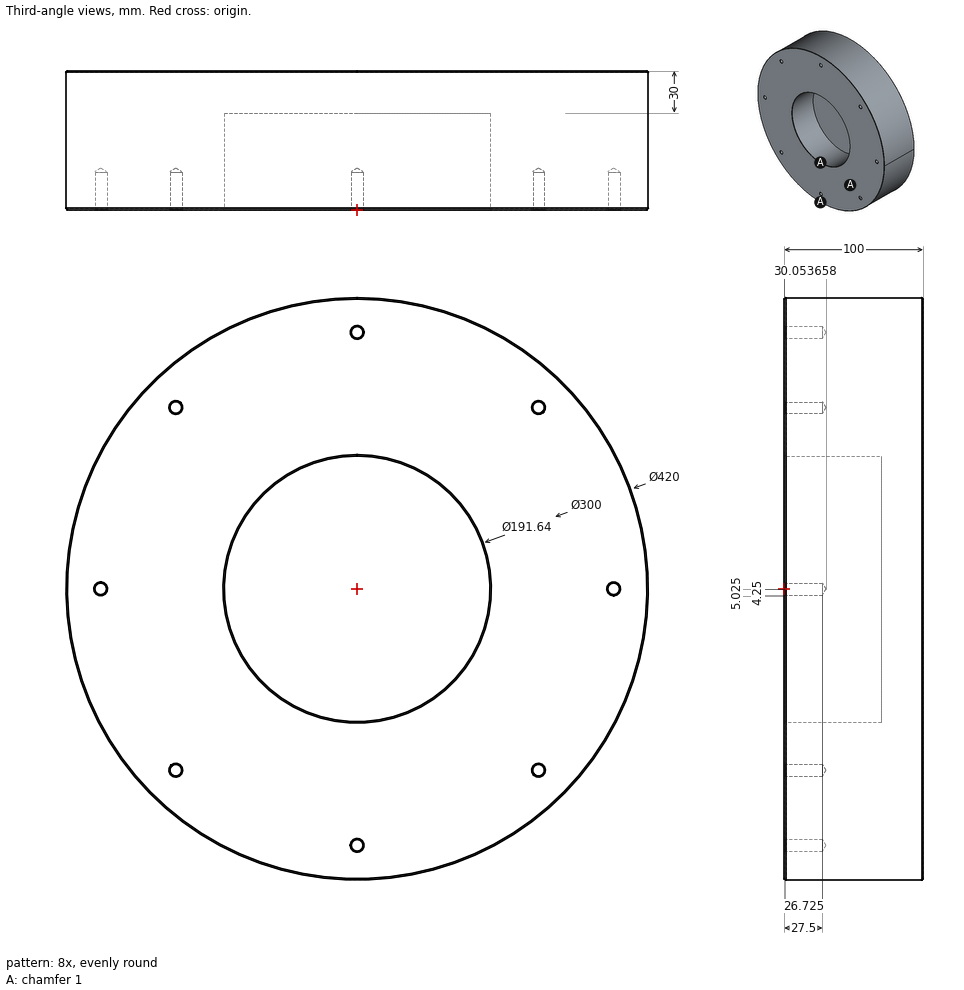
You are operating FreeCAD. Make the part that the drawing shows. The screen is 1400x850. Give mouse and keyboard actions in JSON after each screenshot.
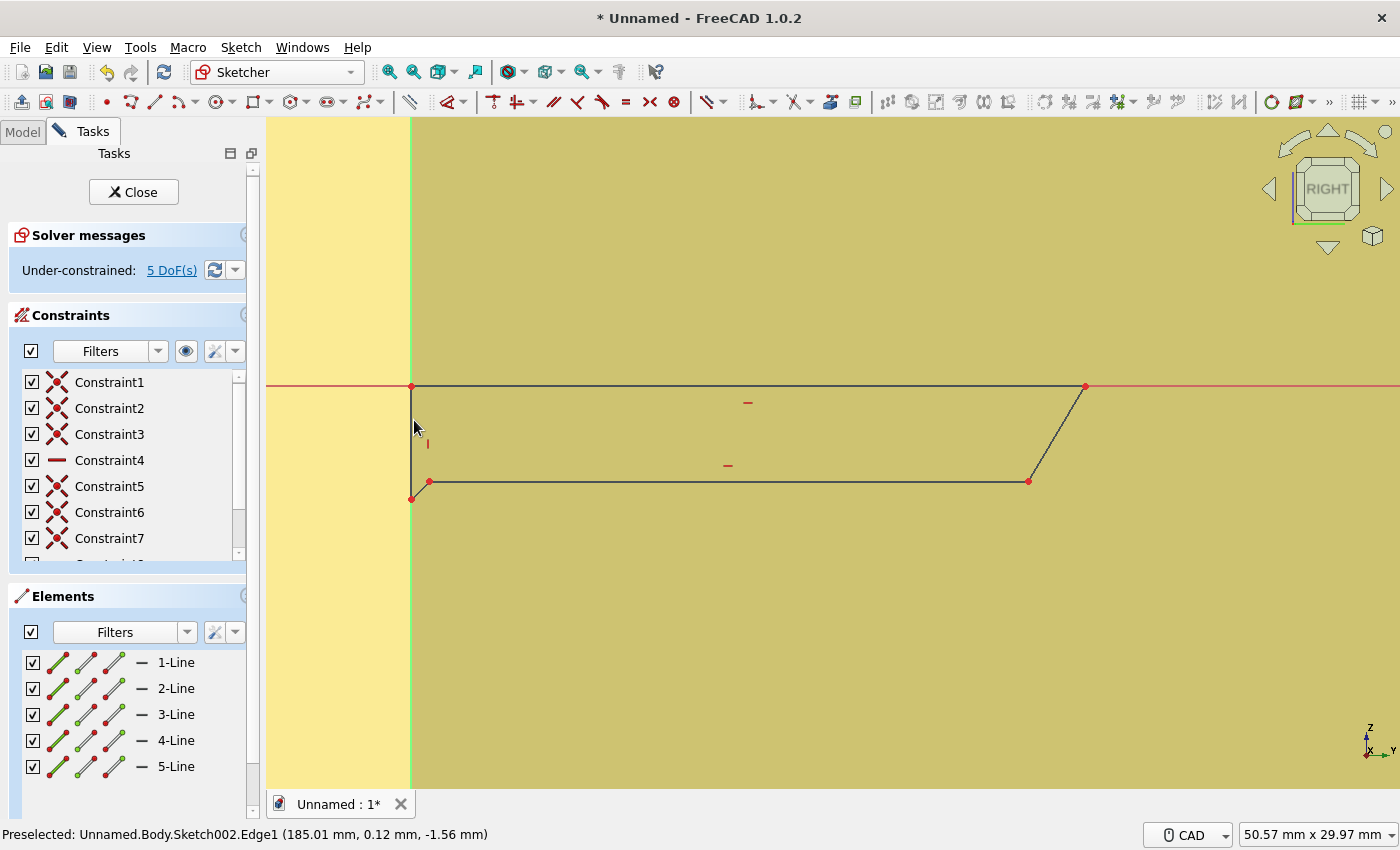
{"action": "left_click", "coordinate": [411, 420]}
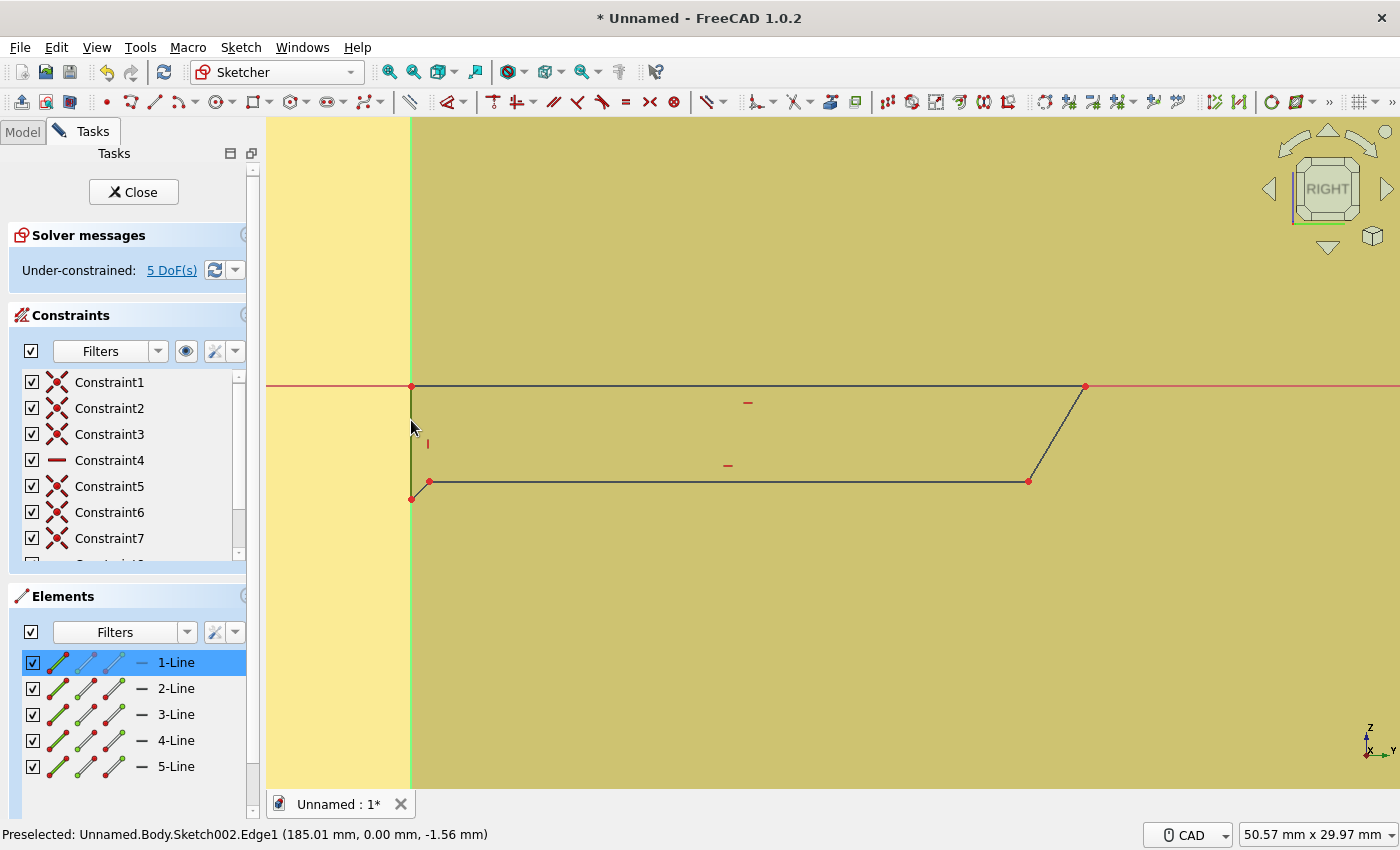
{"action": "left_click", "coordinate": [466, 102]}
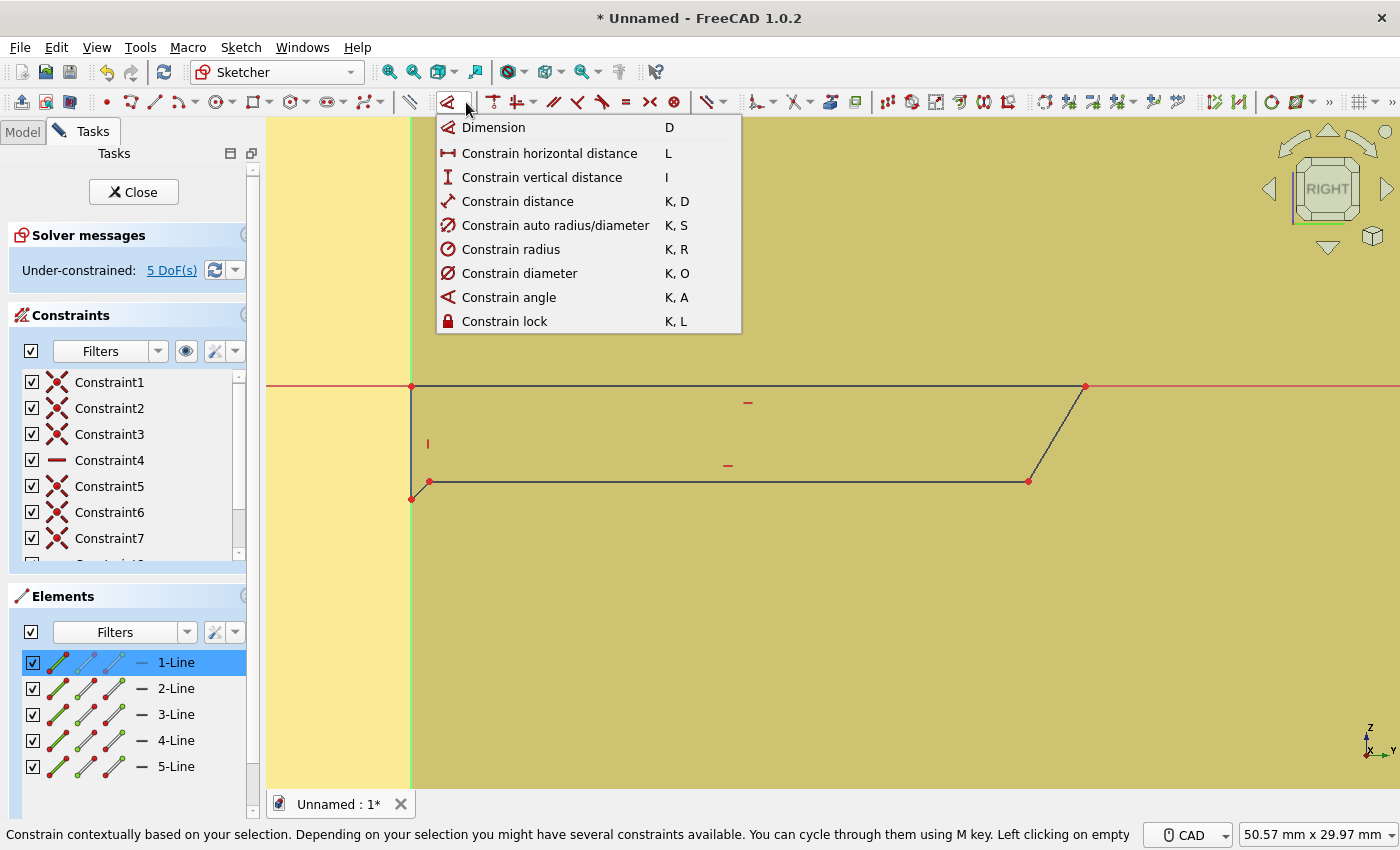
{"action": "left_click", "coordinate": [589, 177]}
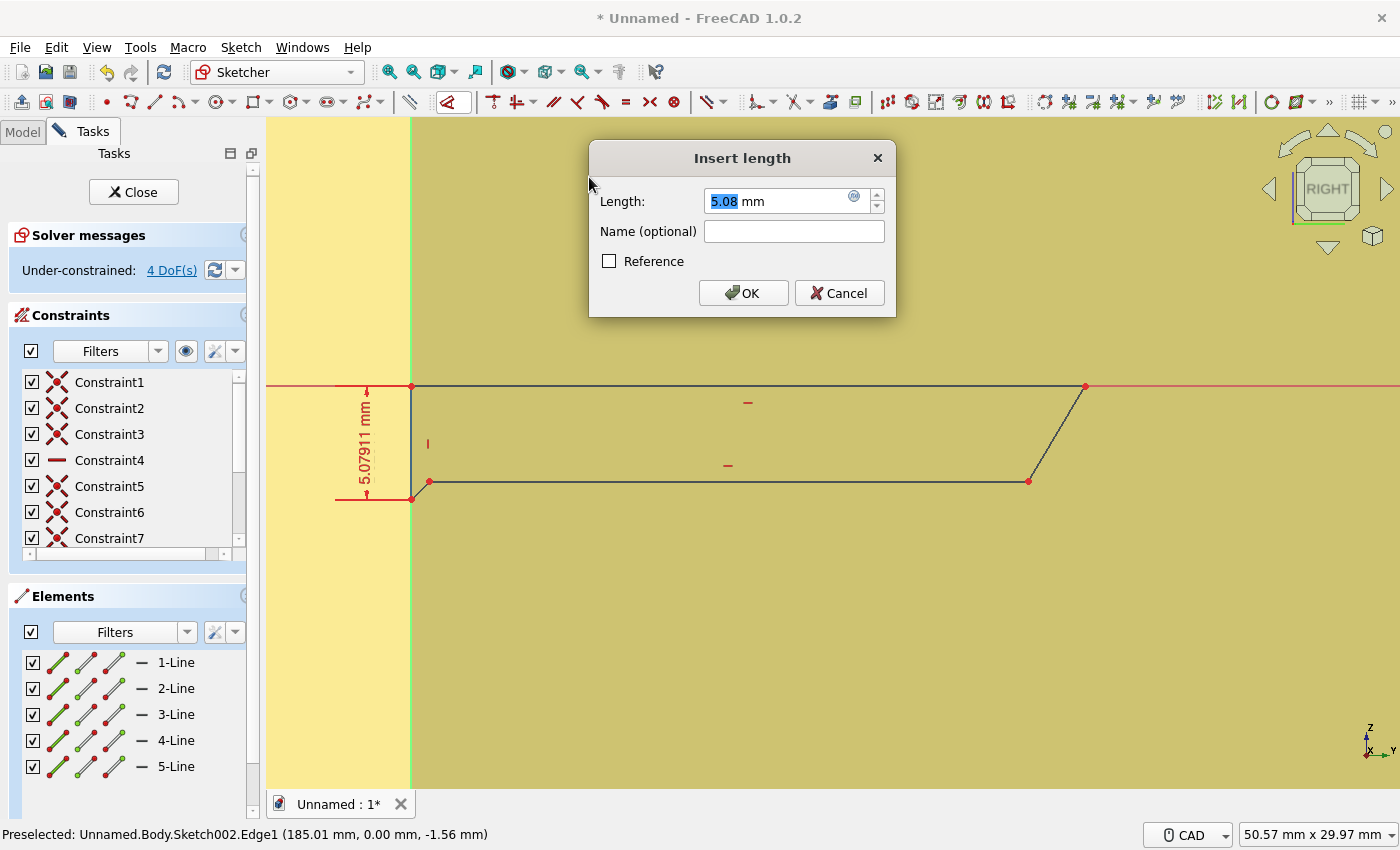
{"action": "type", "text": "5.025"}
{"action": "key", "text": "Return"}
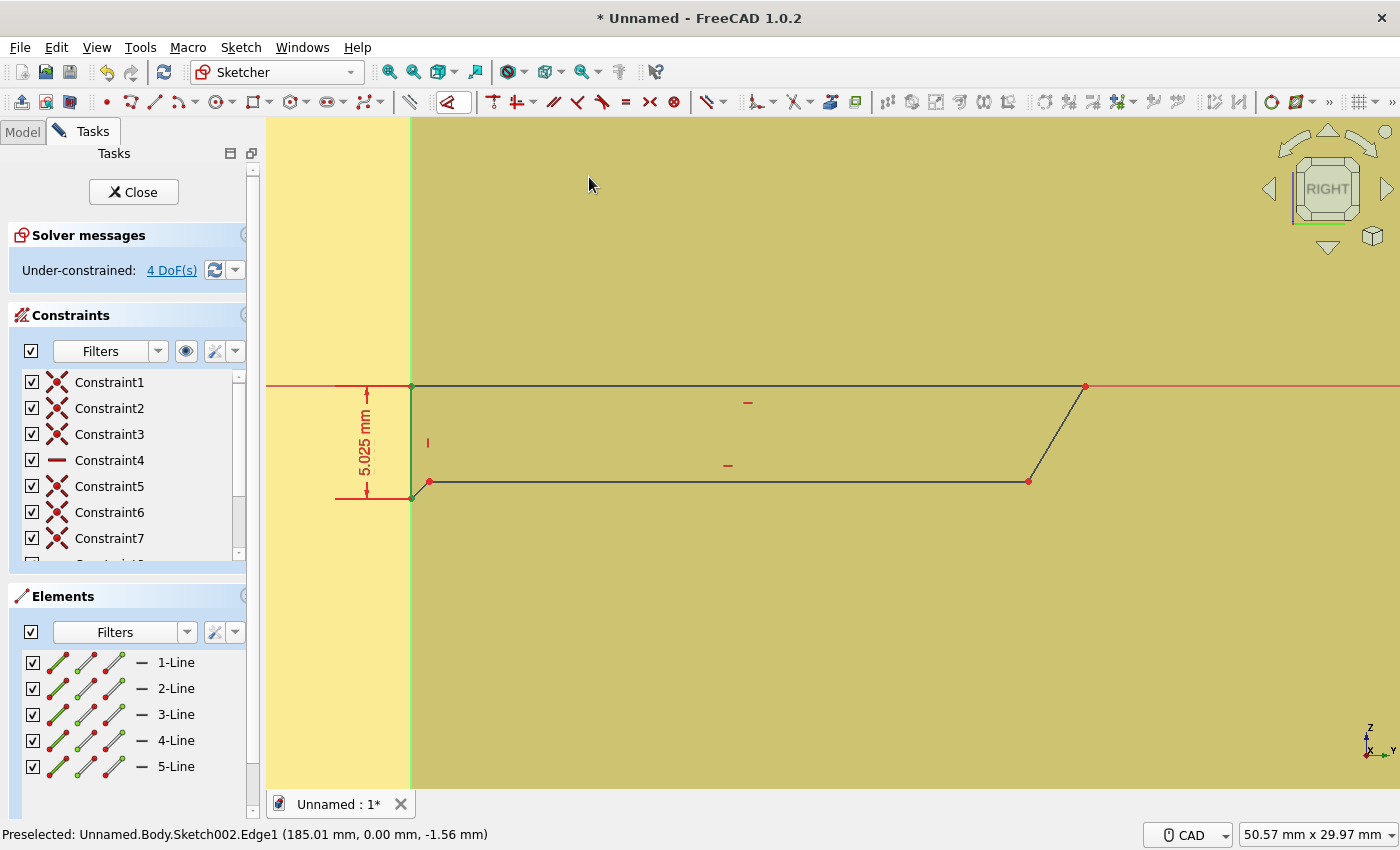
{"action": "left_click", "coordinate": [429, 482]}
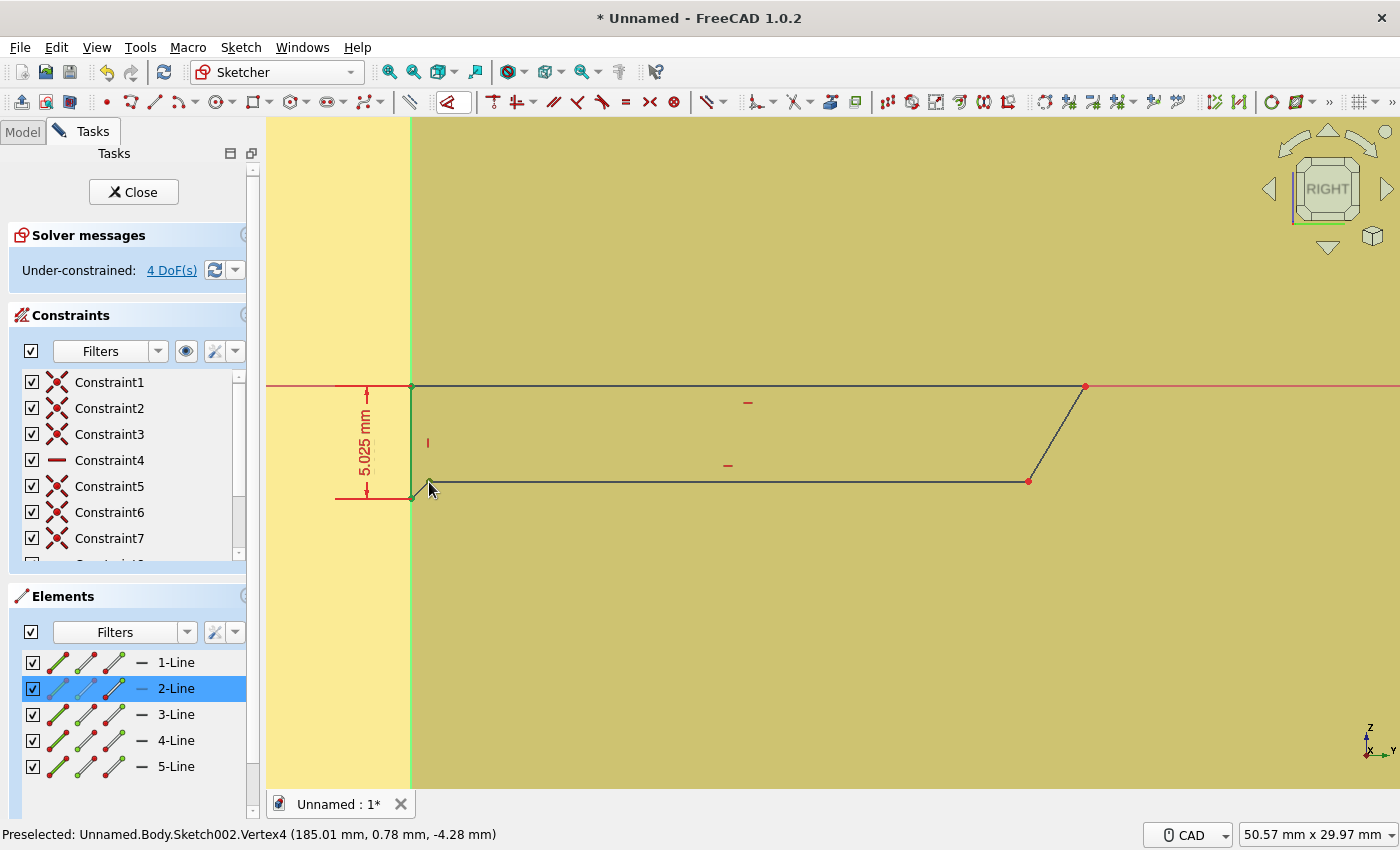
{"action": "key", "text": "i"}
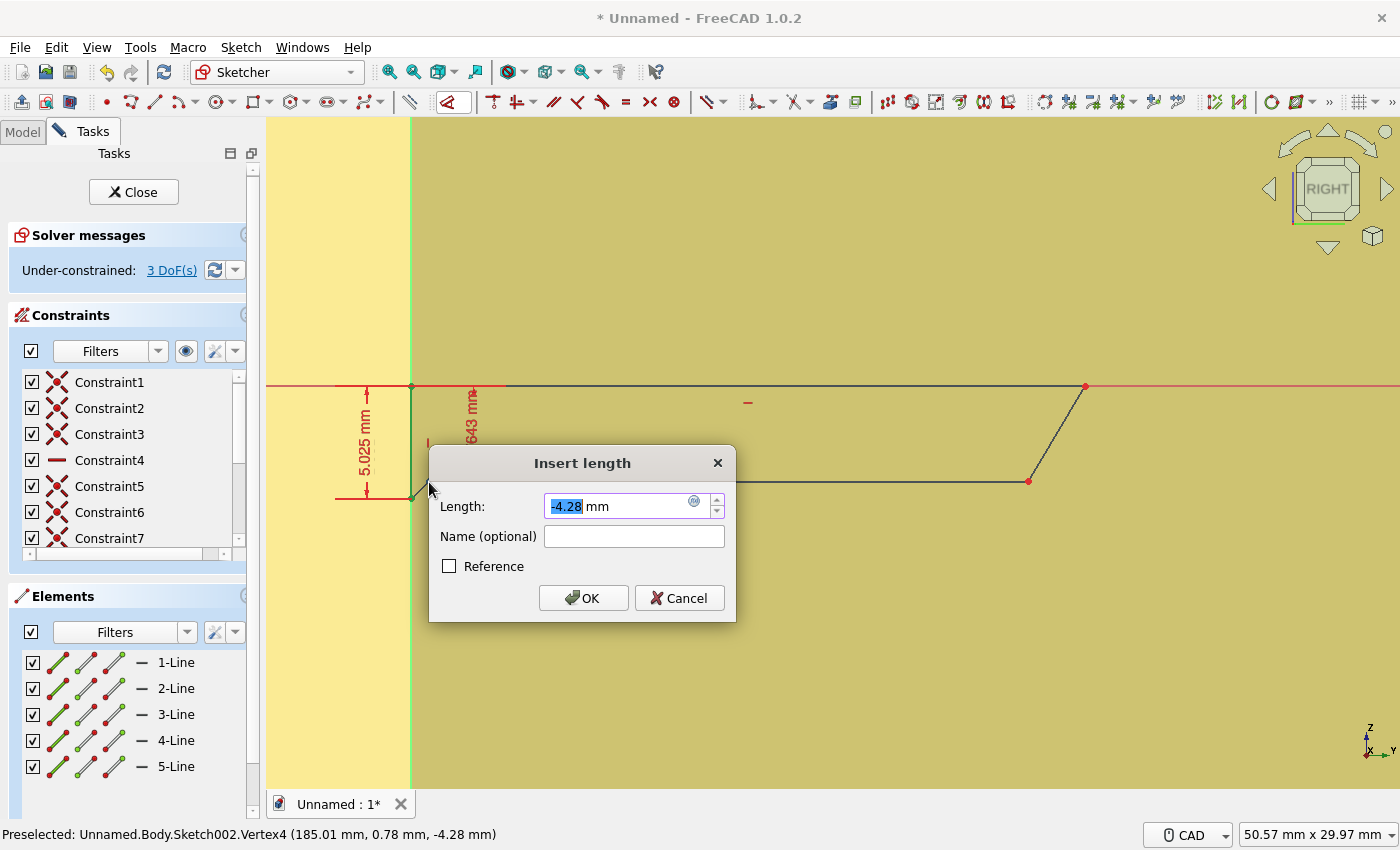
{"action": "type", "text": "-4.25"}
{"action": "key", "text": "Return"}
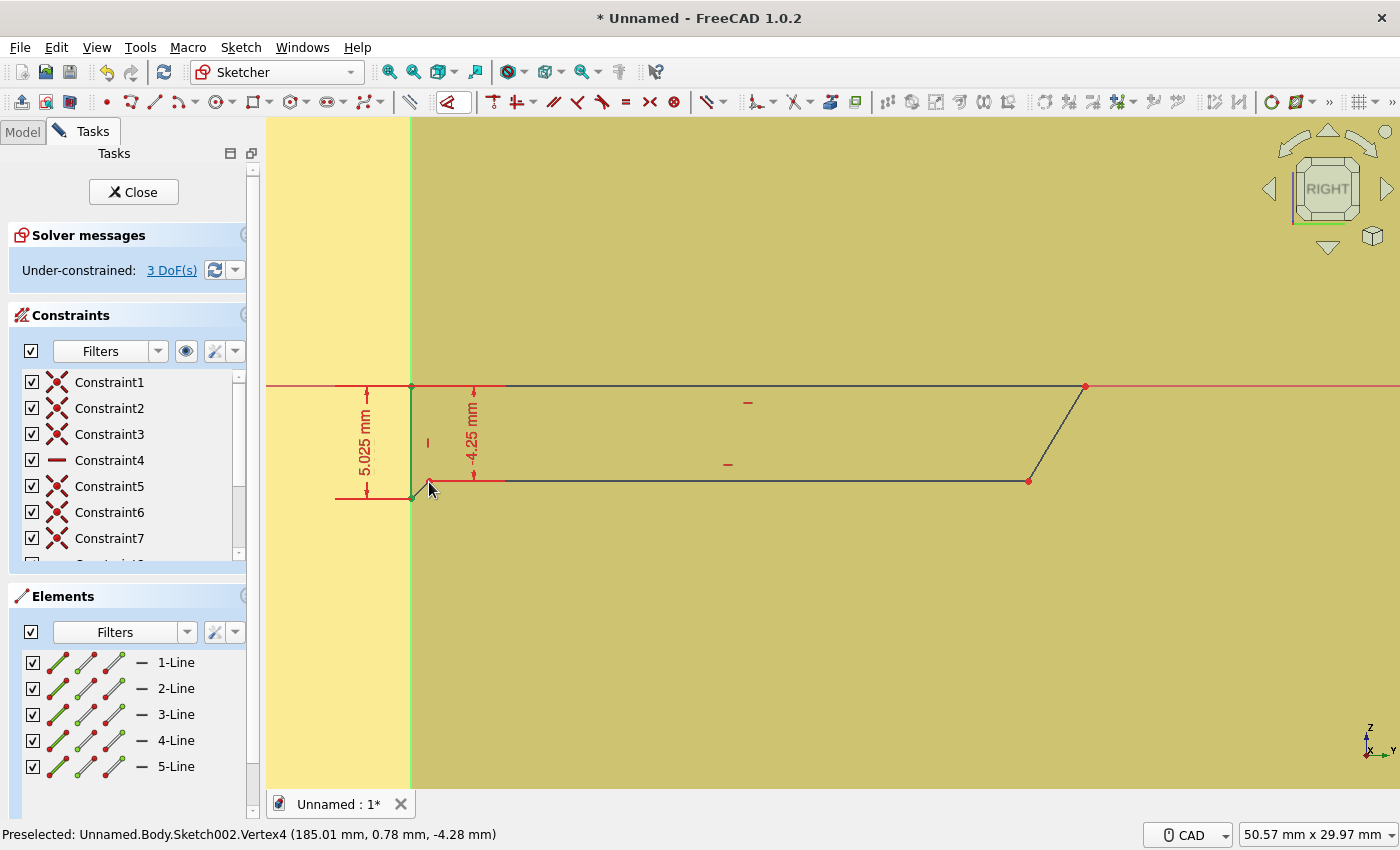
{"action": "left_click", "coordinate": [1028, 481]}